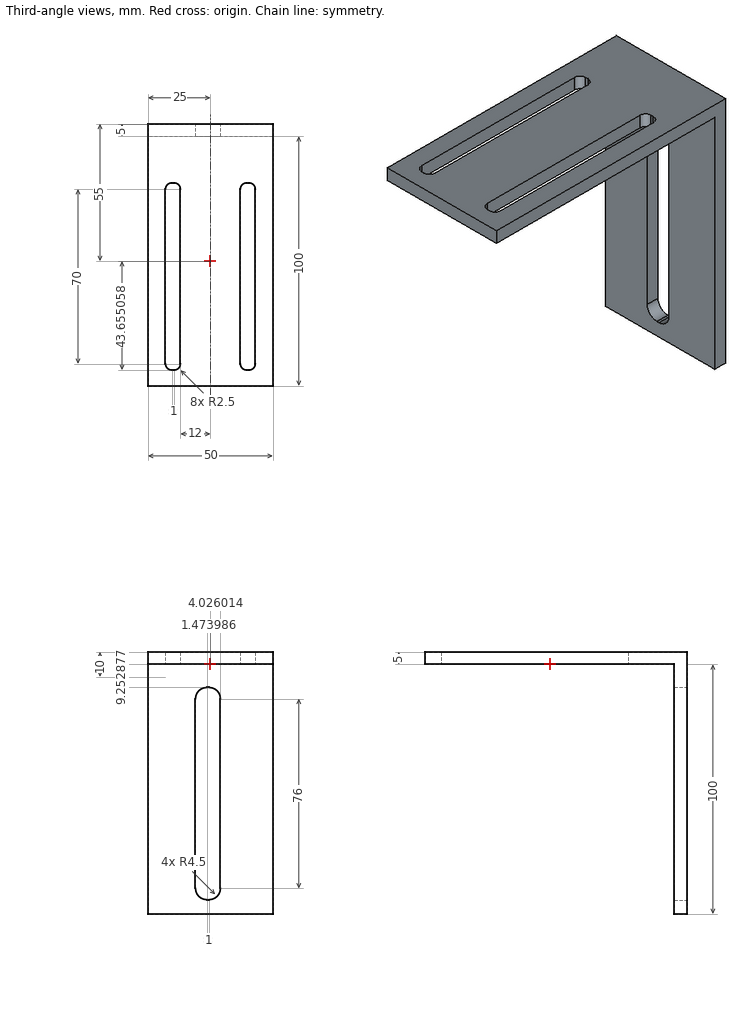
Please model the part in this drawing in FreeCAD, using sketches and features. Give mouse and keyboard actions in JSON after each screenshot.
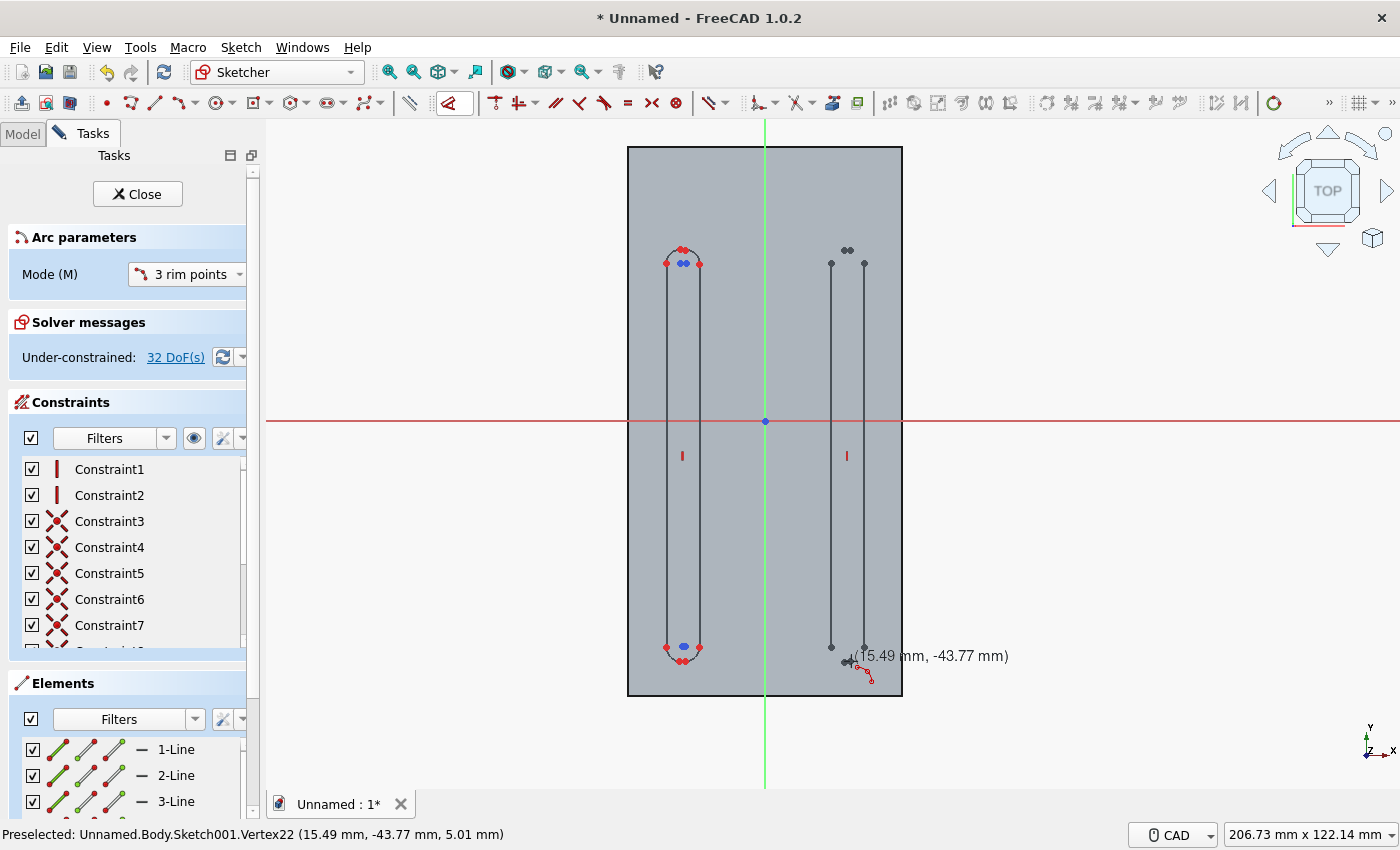
{"action": "left_click", "coordinate": [864, 647]}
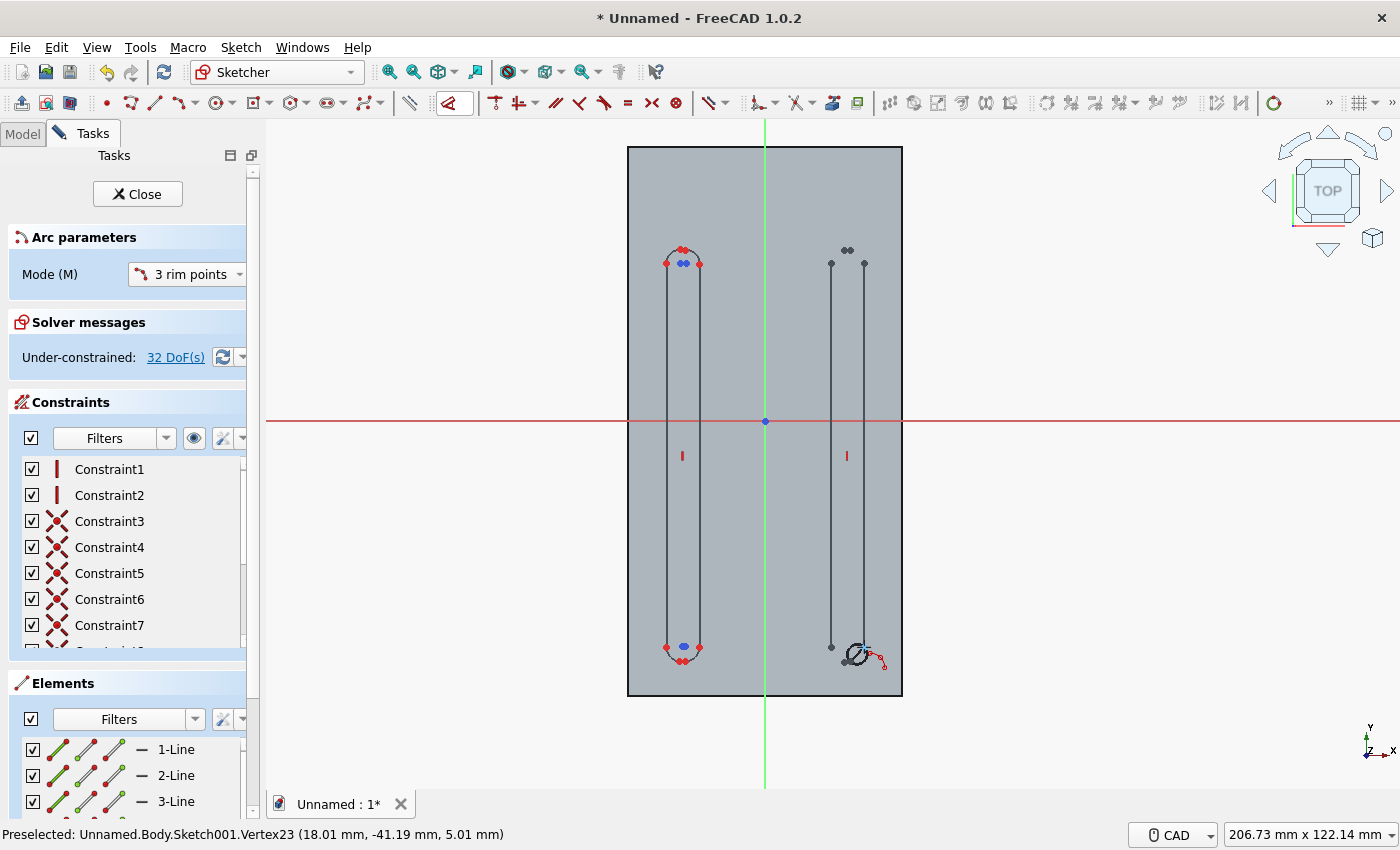
{"action": "scroll", "coordinate": [860, 657], "scroll_direction": "up", "scroll_amount": 7}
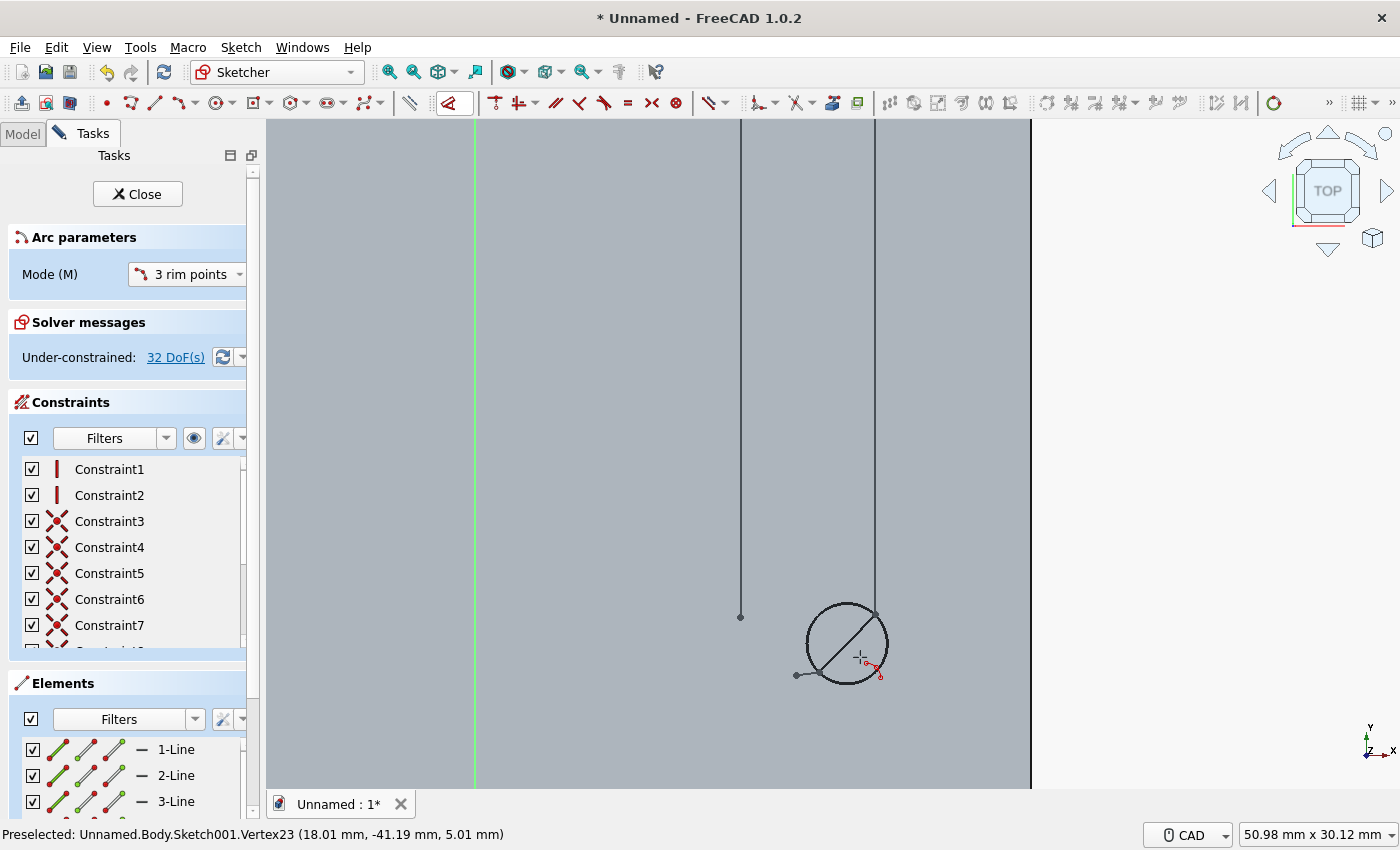
{"action": "left_click", "coordinate": [859, 654]}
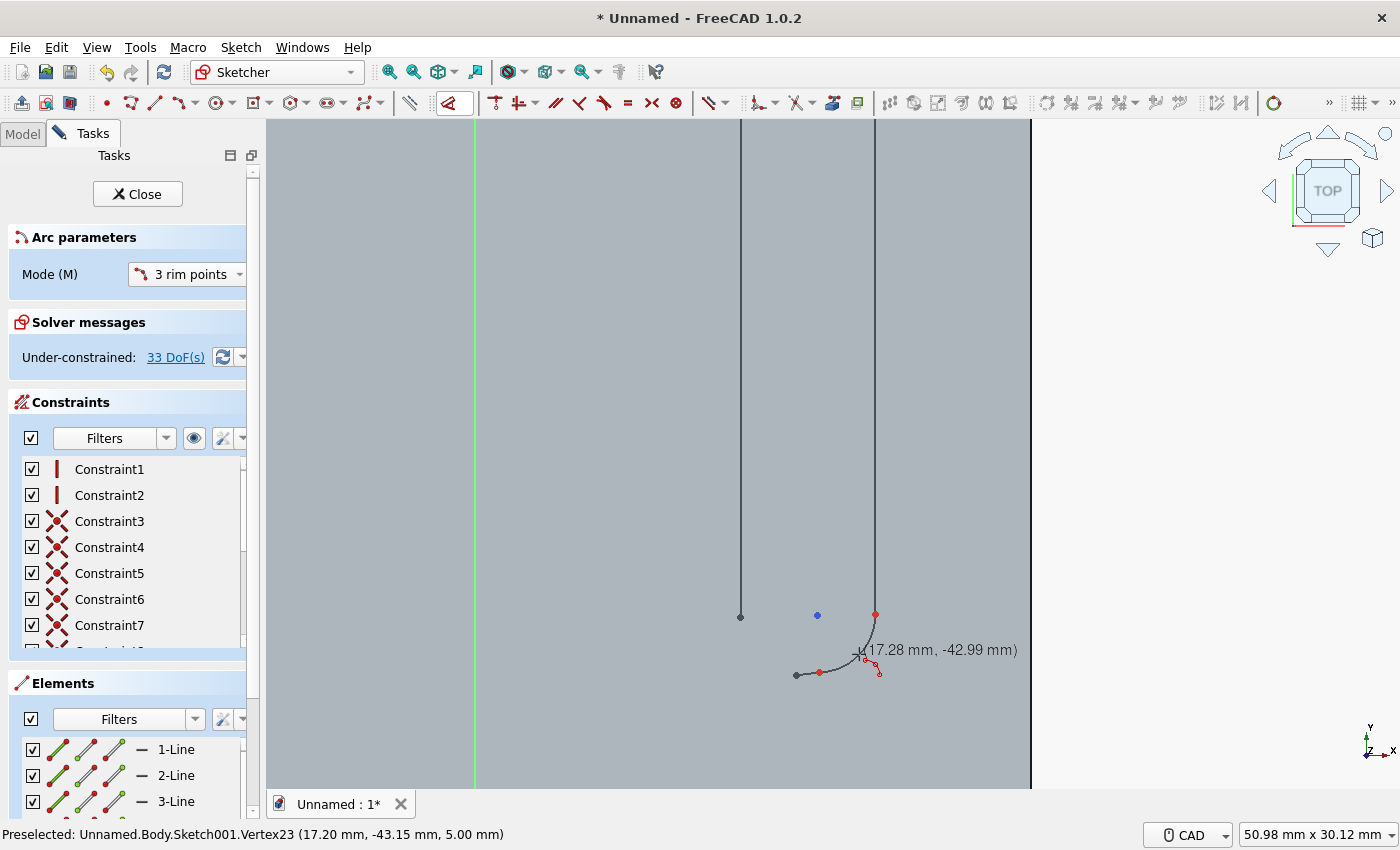
{"action": "scroll", "coordinate": [859, 656], "scroll_direction": "down", "scroll_amount": 7}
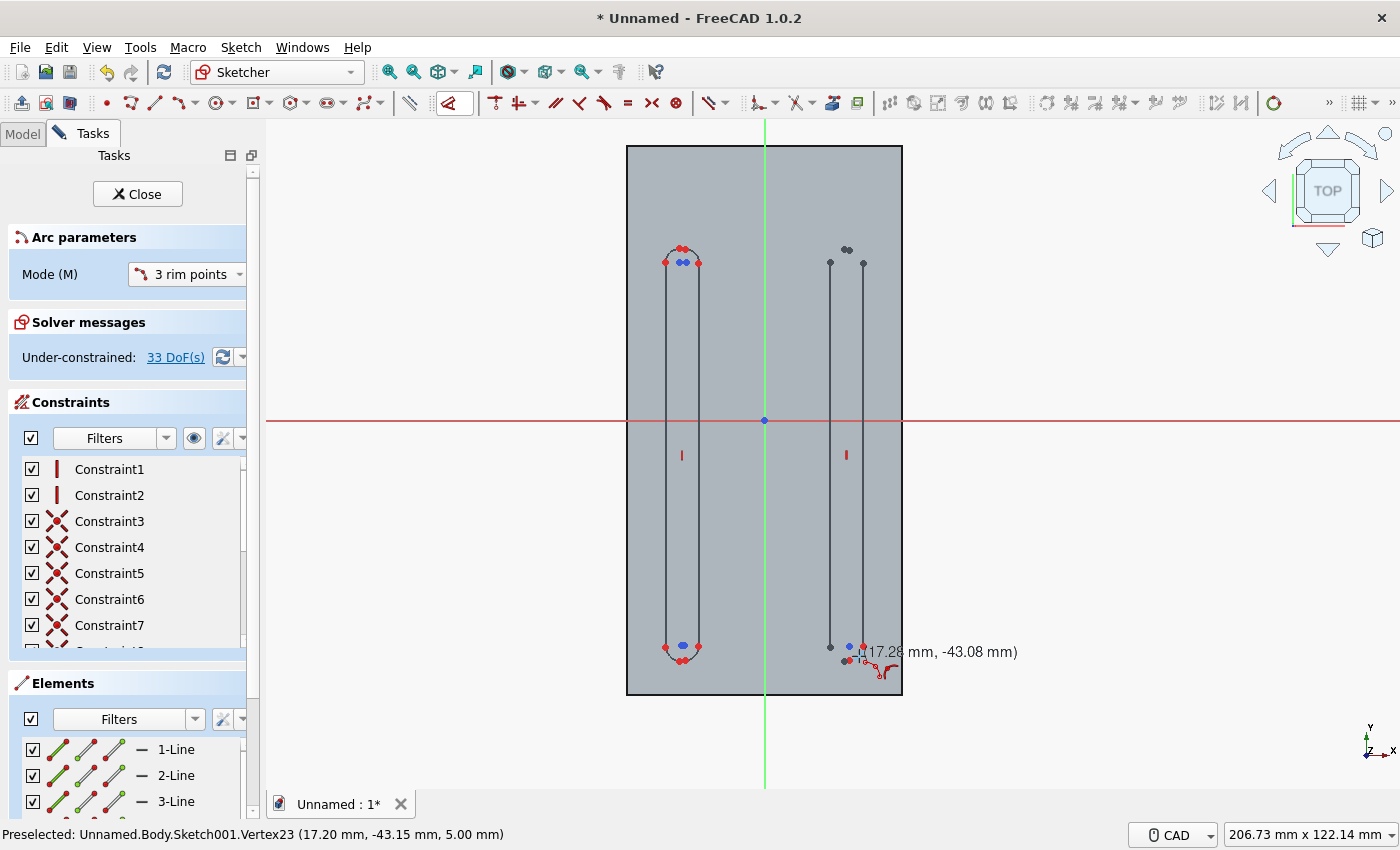
{"action": "left_click", "coordinate": [863, 263]}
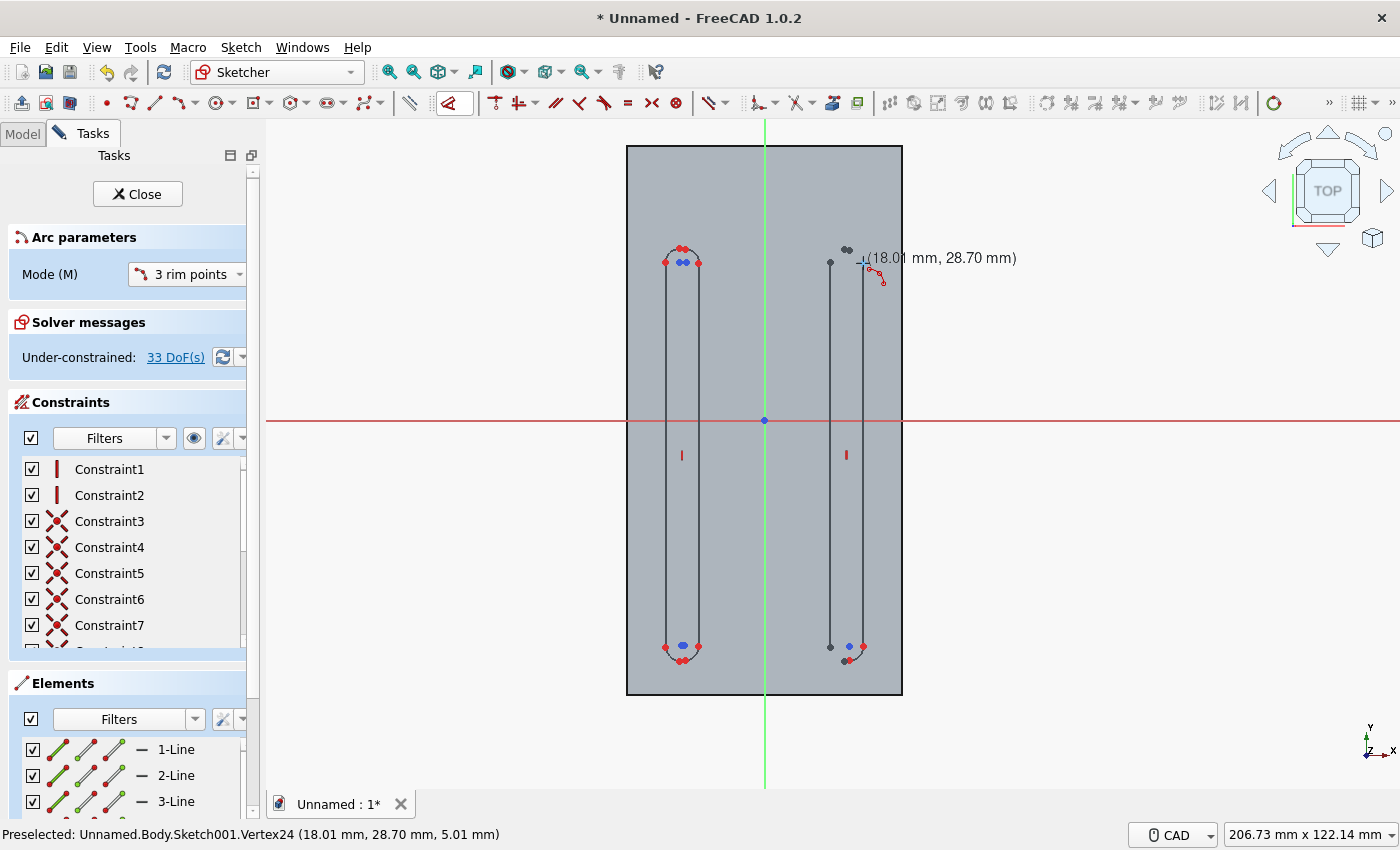
{"action": "scroll", "coordinate": [850, 249], "scroll_direction": "up", "scroll_amount": 9}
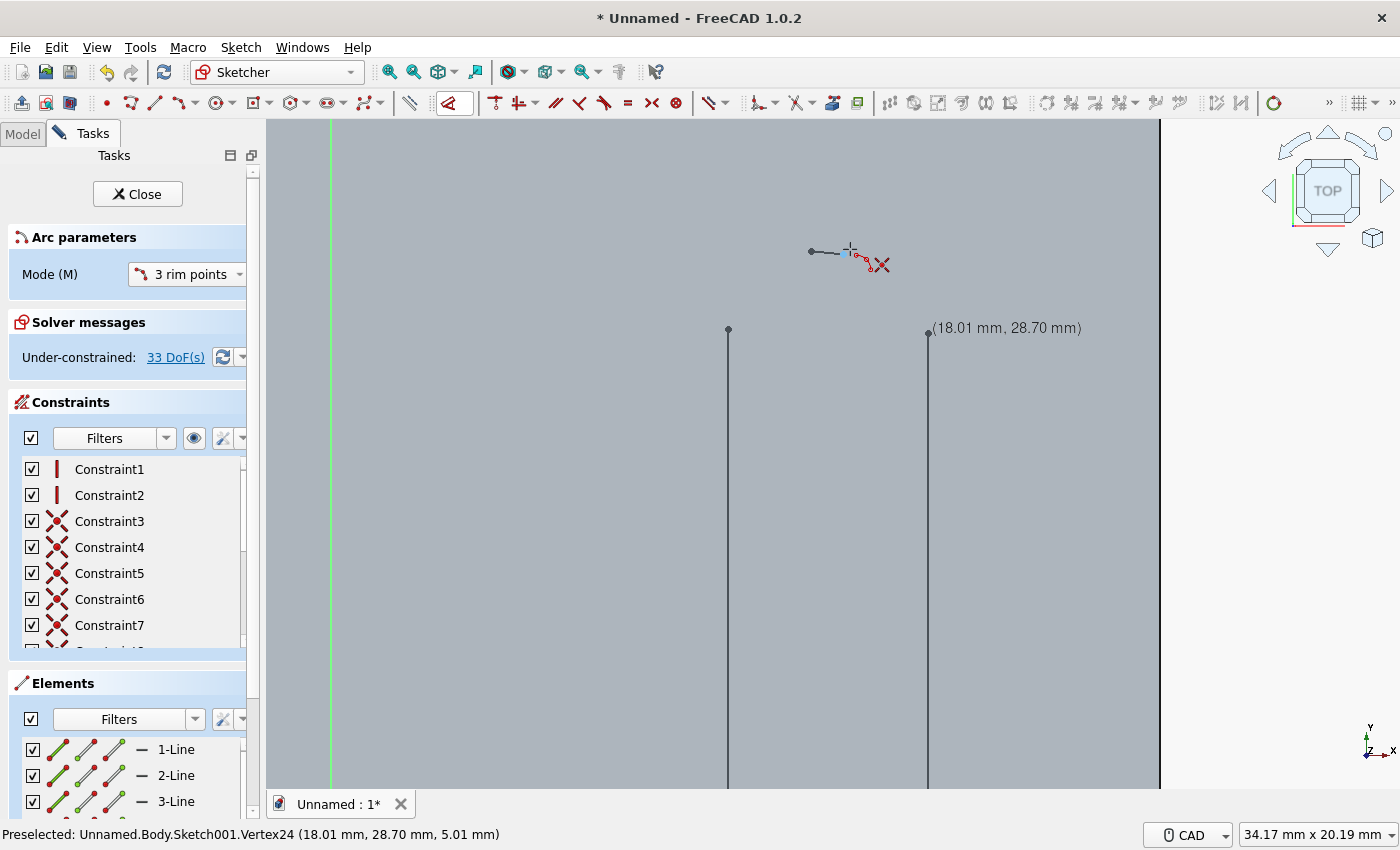
{"action": "left_click", "coordinate": [844, 255]}
{"action": "left_click", "coordinate": [904, 270]}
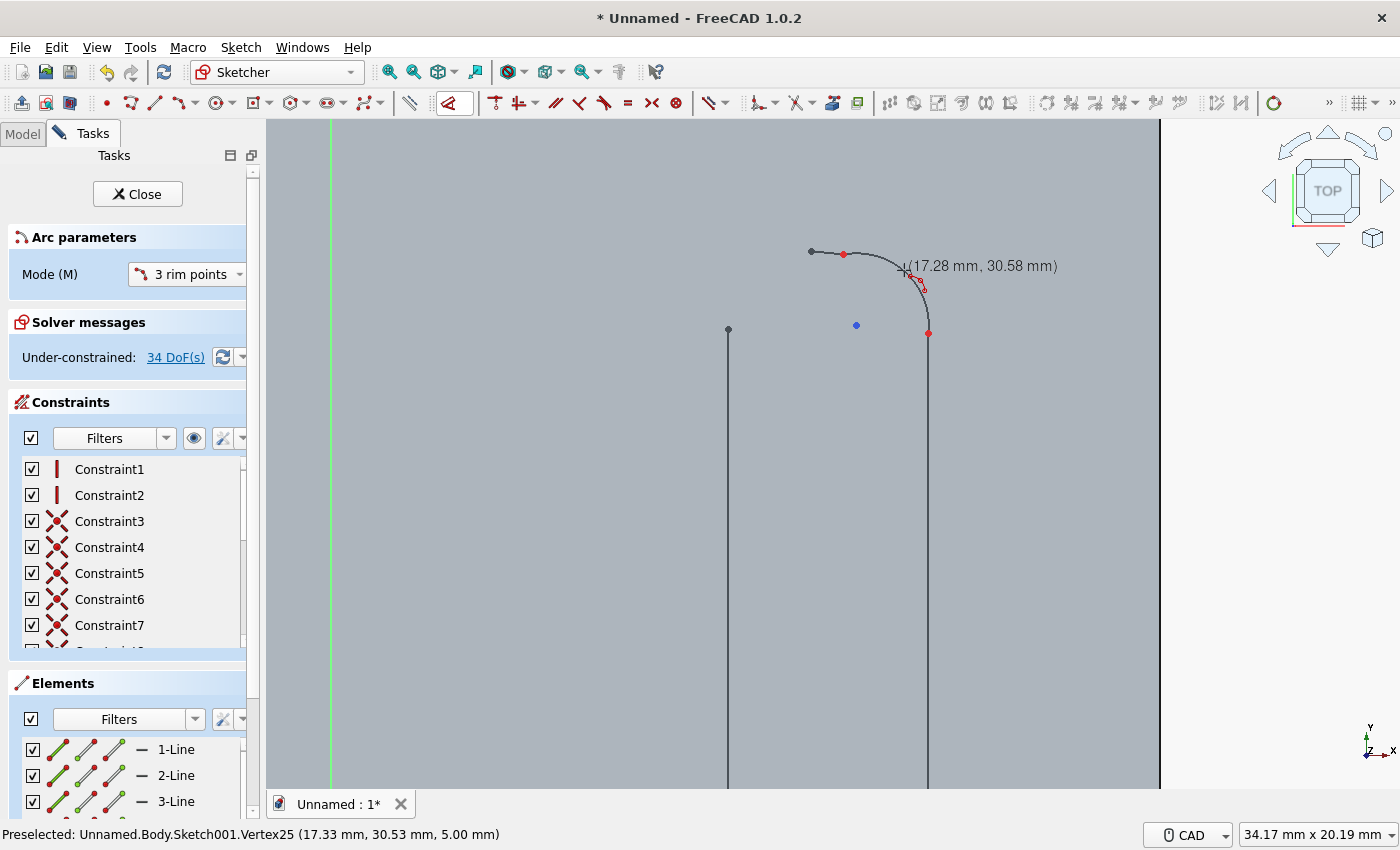
{"action": "left_click", "coordinate": [812, 251]}